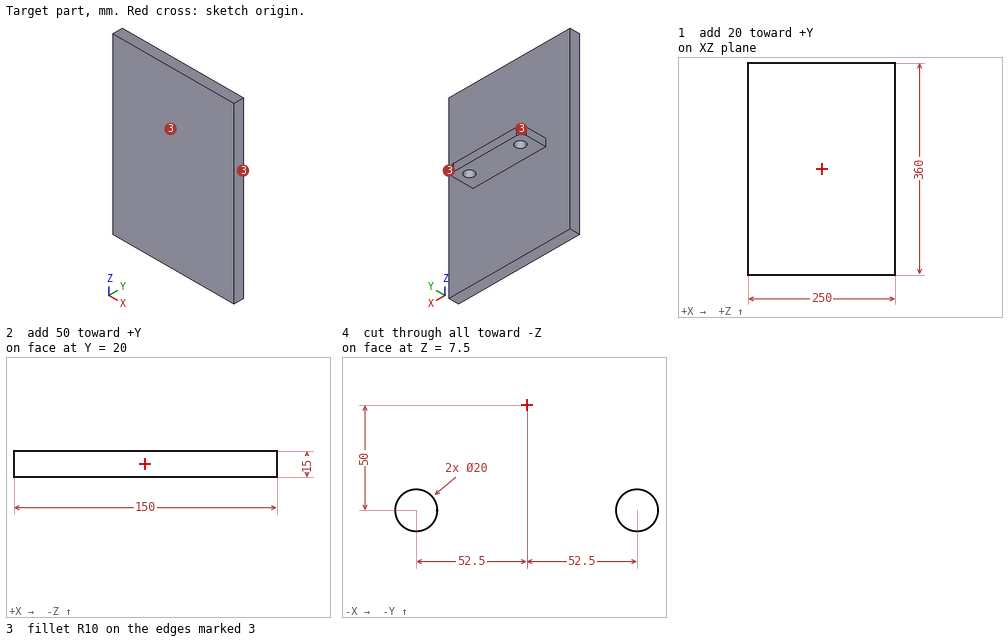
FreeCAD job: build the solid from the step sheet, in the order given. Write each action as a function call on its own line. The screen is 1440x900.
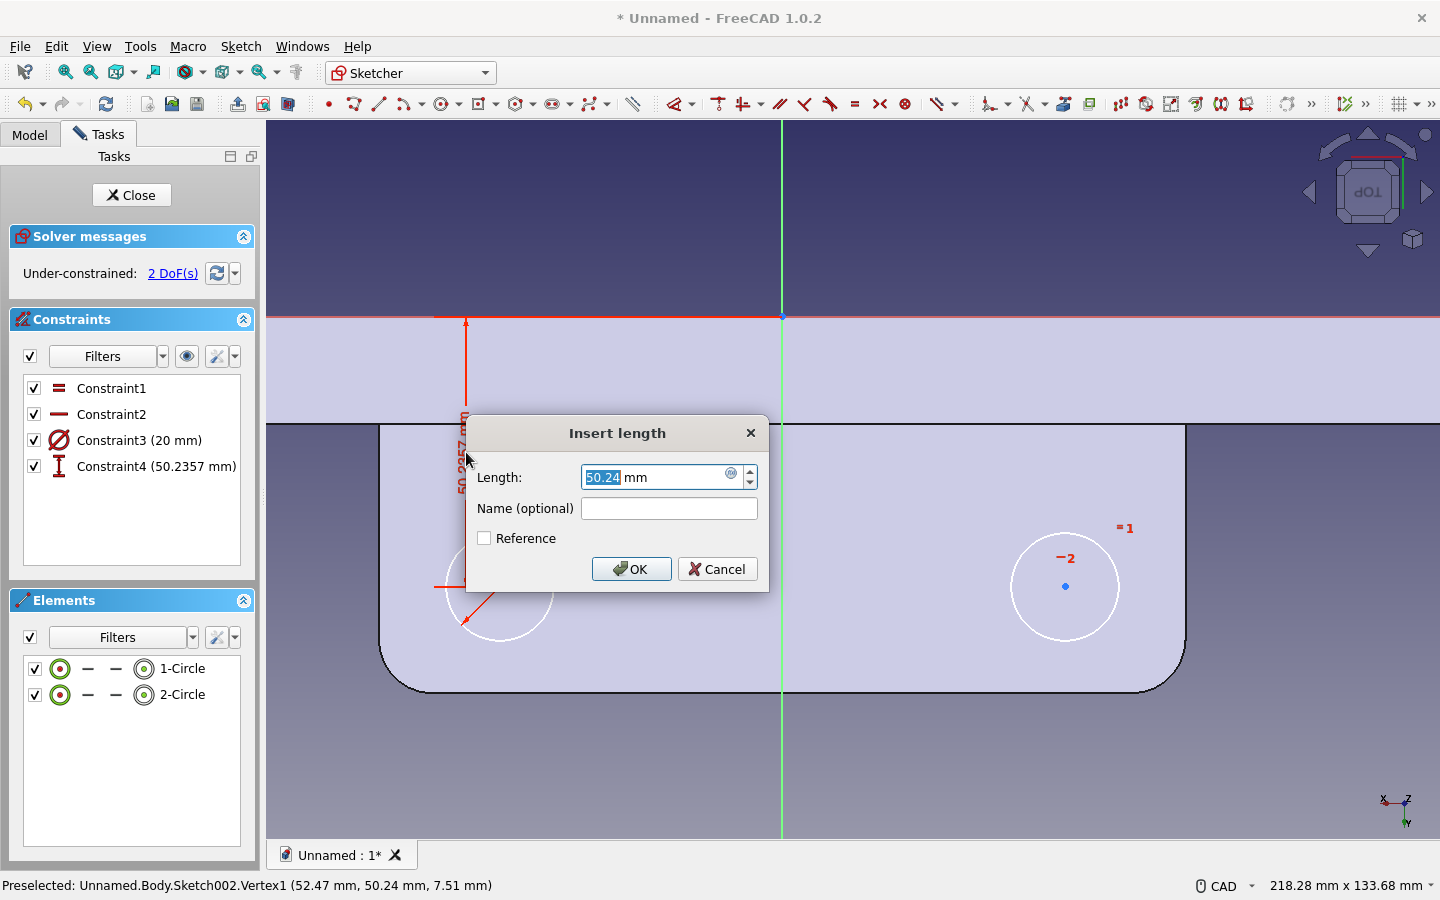
text(50)
key(Return)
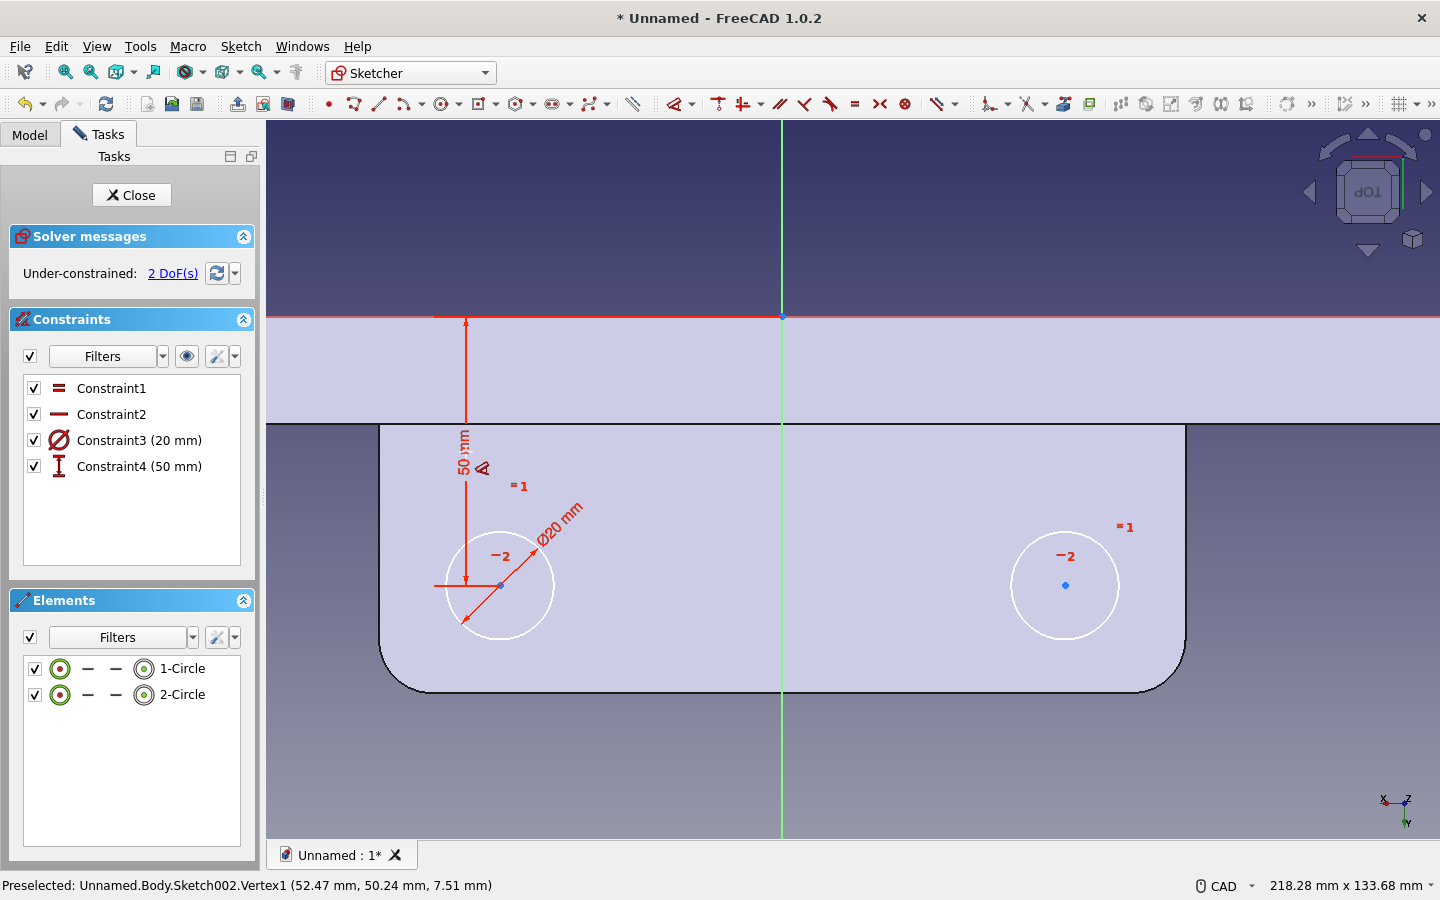
click(500, 586)
click(641, 283)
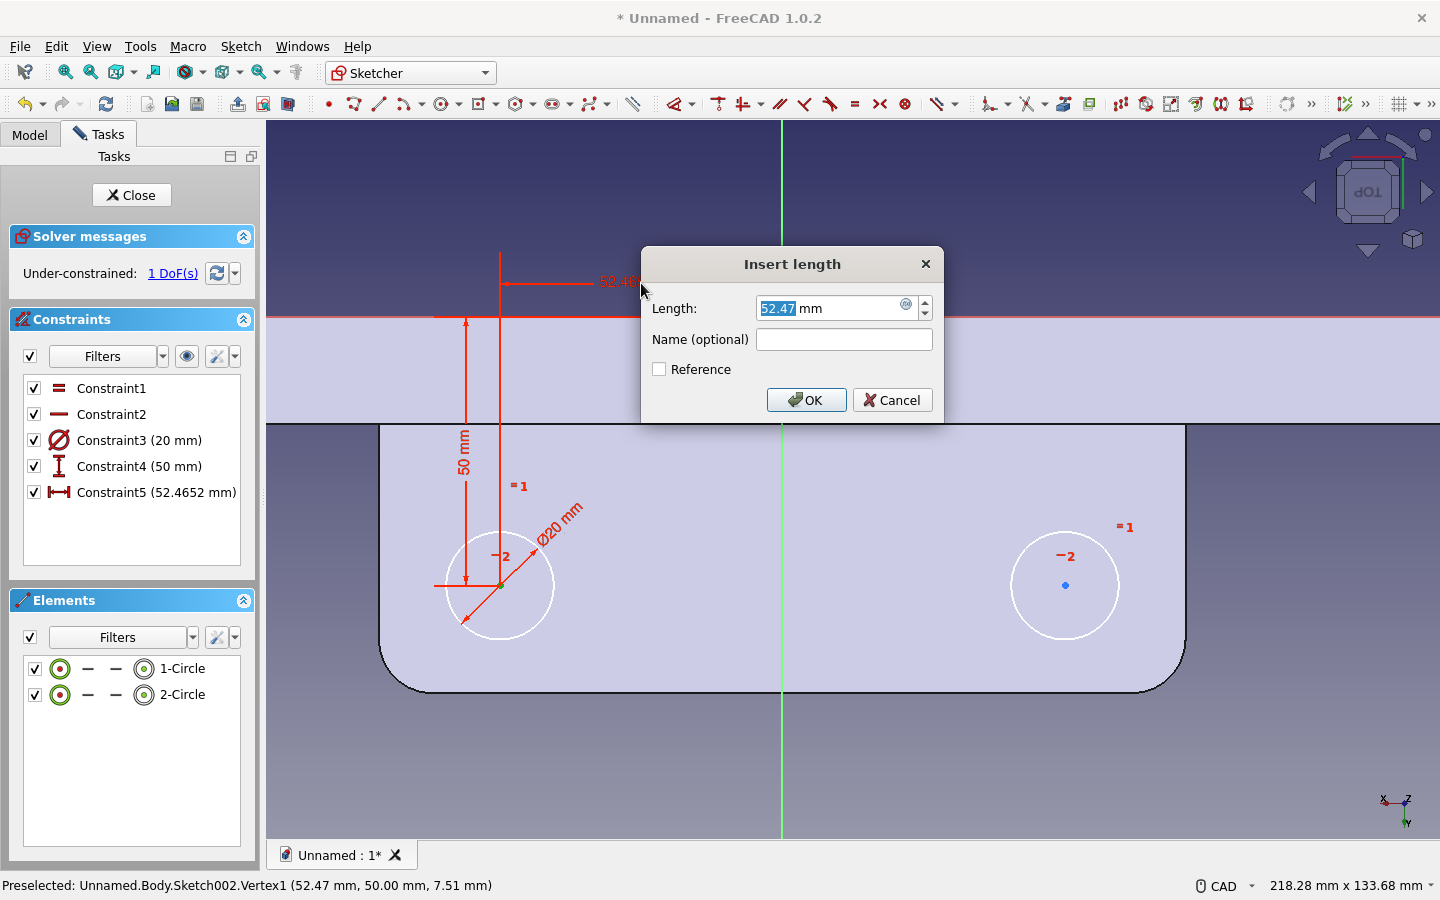
text(52.5)
key(Return)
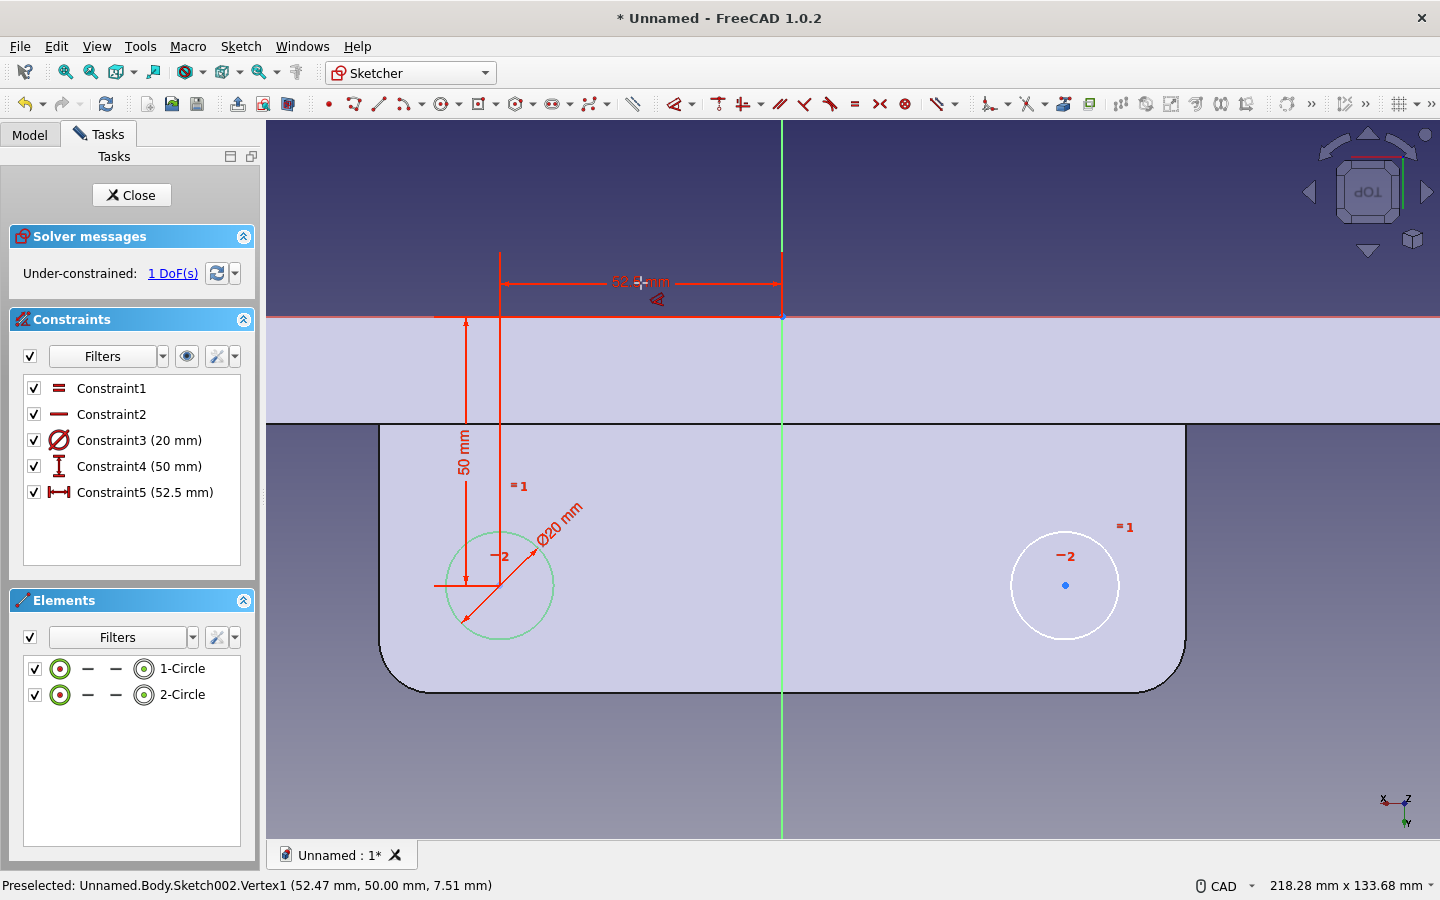
click(1065, 586)
click(924, 283)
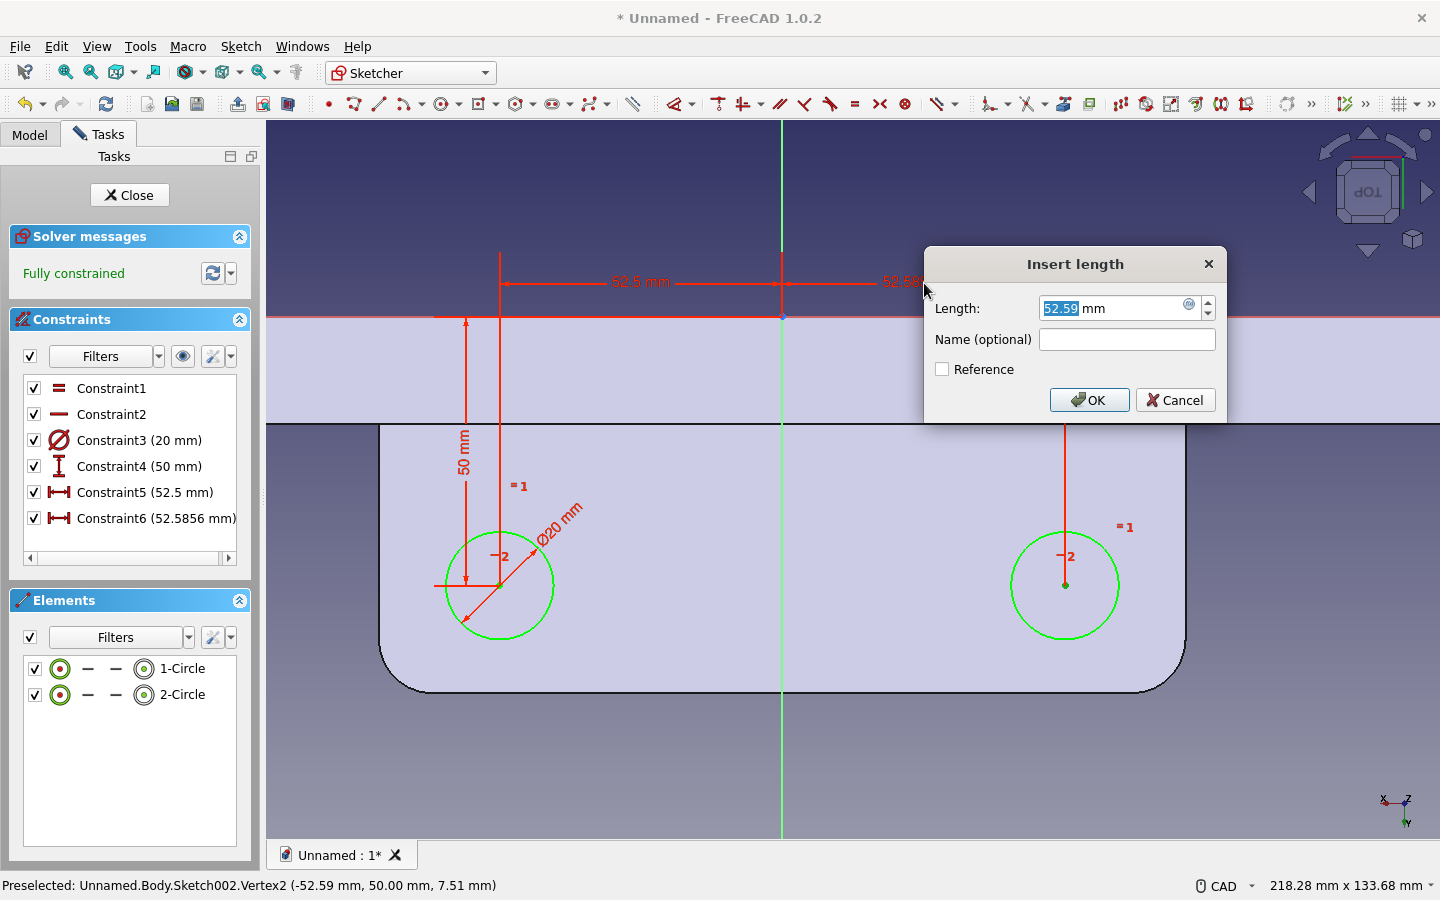
text(52.5)
key(Return)
key(Escape)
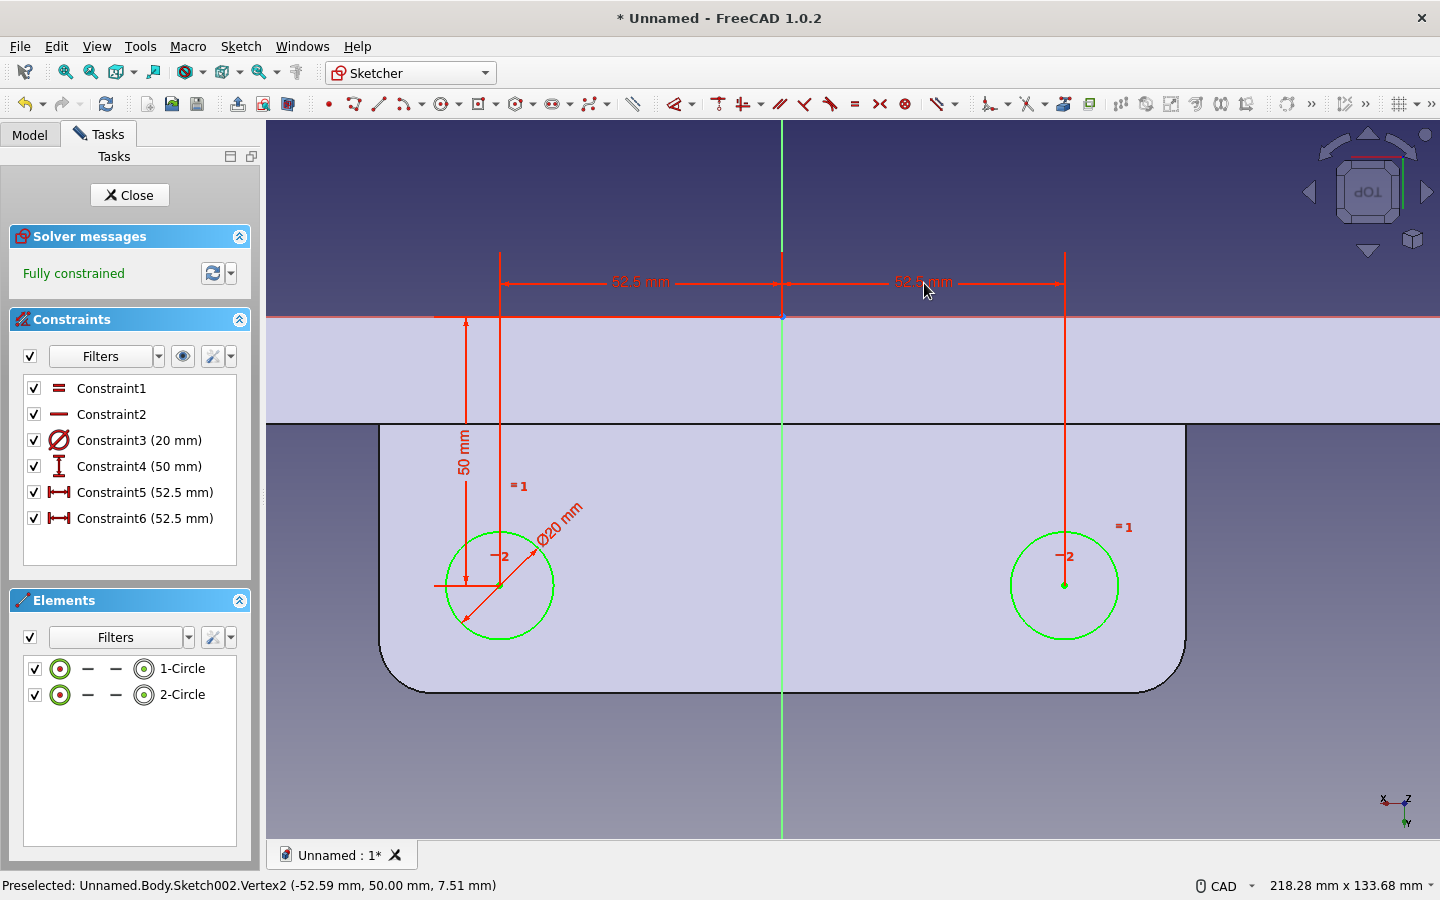
click(130, 195)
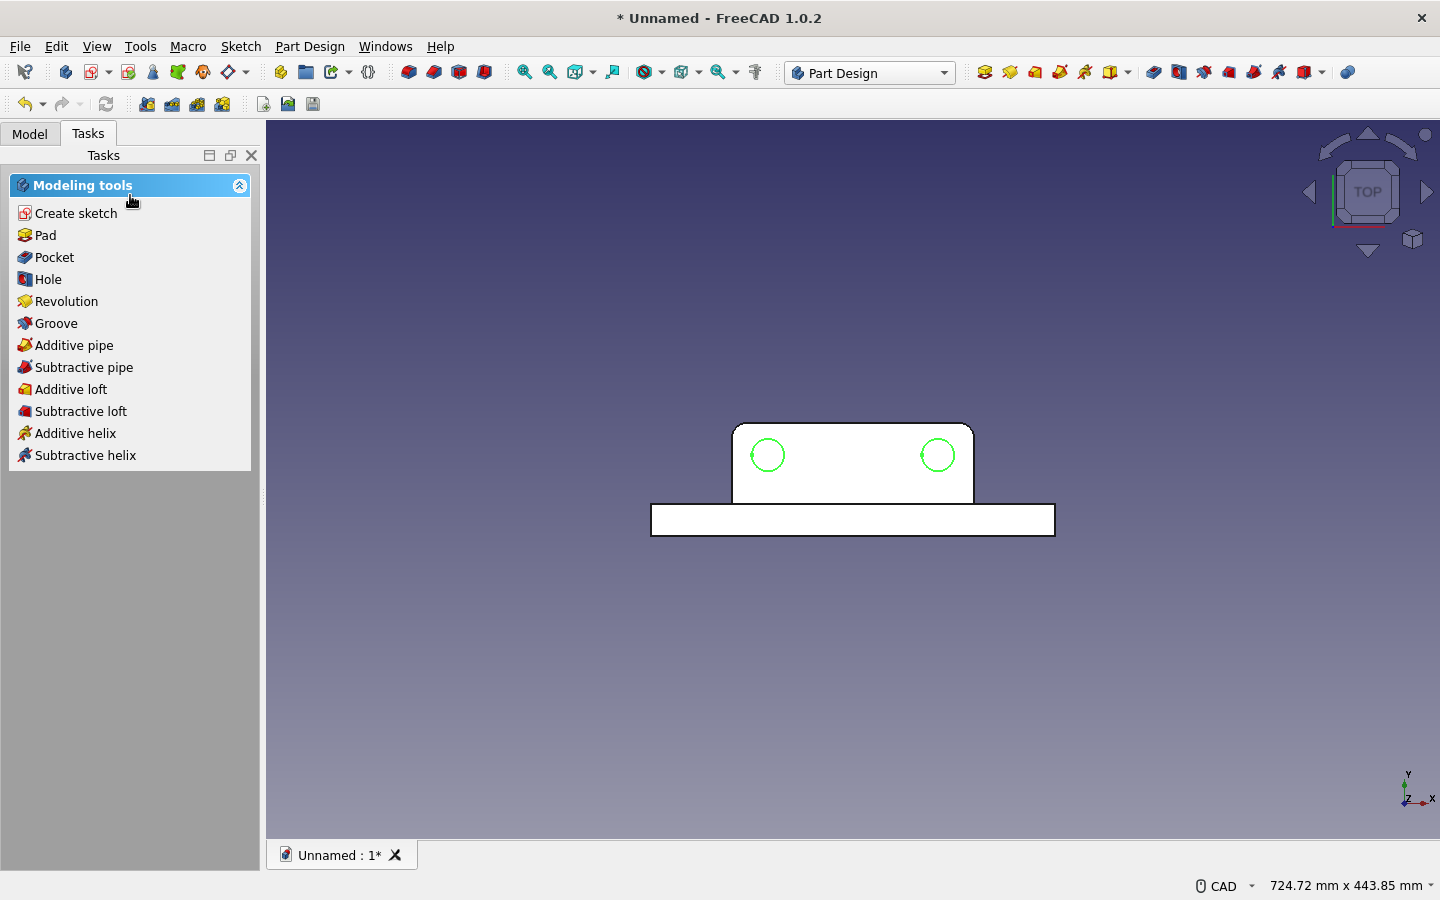
click(1154, 72)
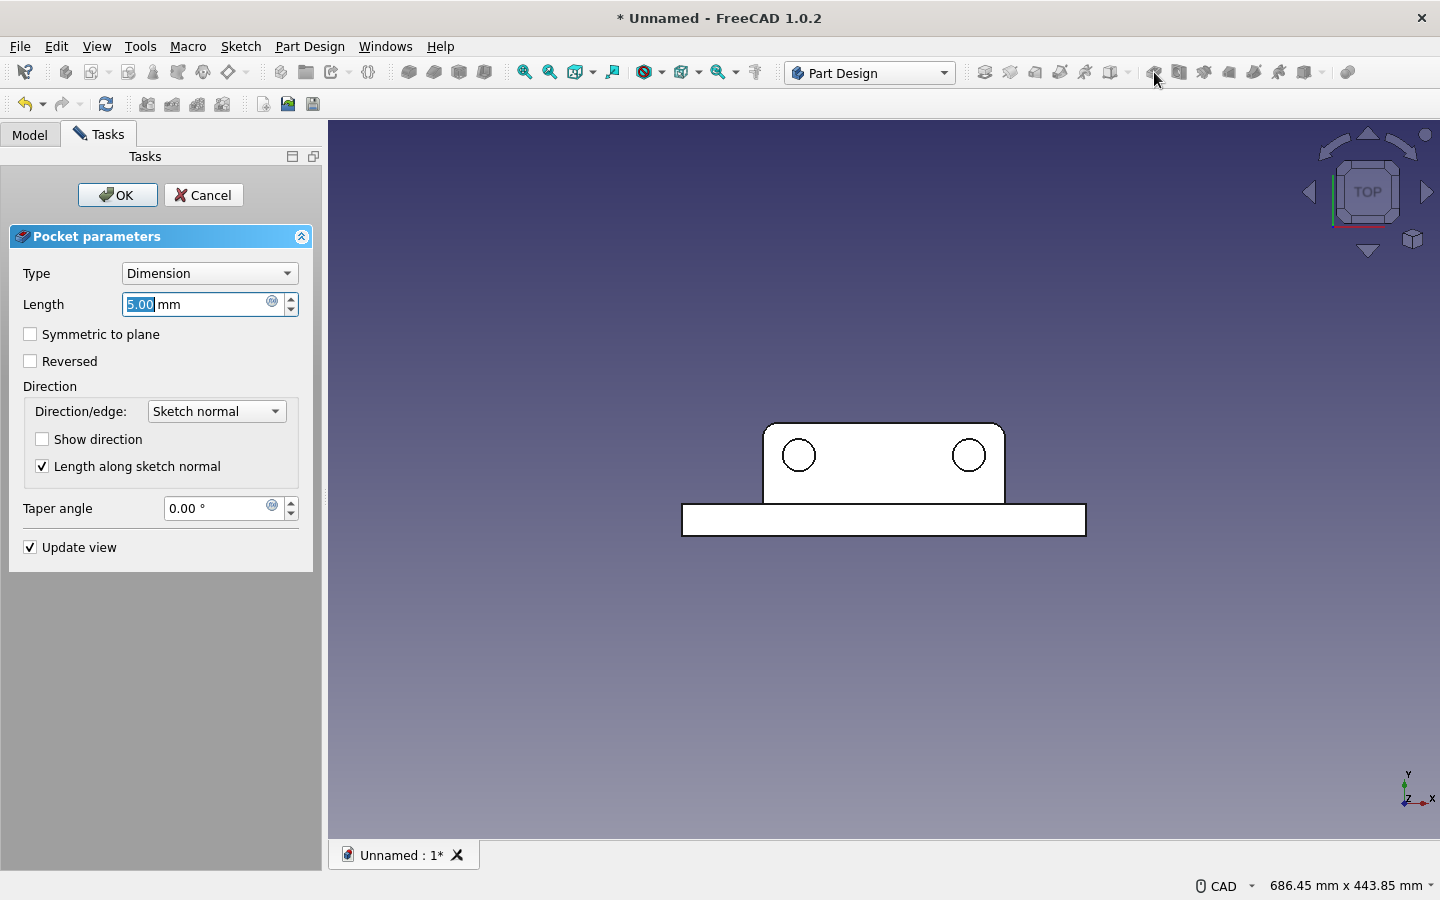
click(210, 274)